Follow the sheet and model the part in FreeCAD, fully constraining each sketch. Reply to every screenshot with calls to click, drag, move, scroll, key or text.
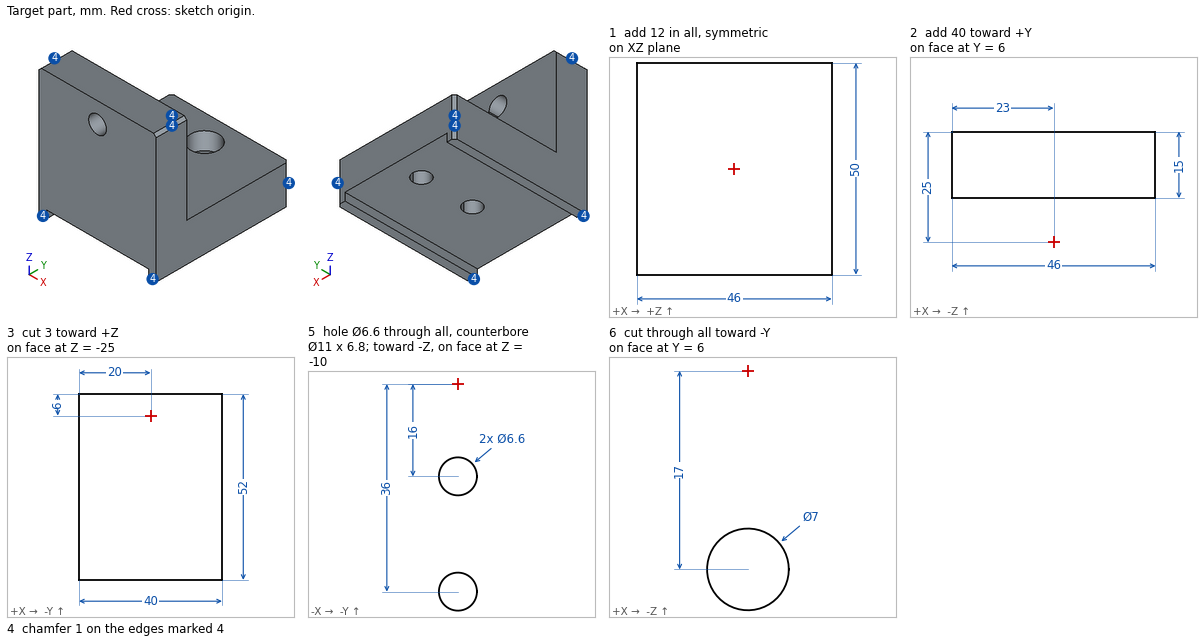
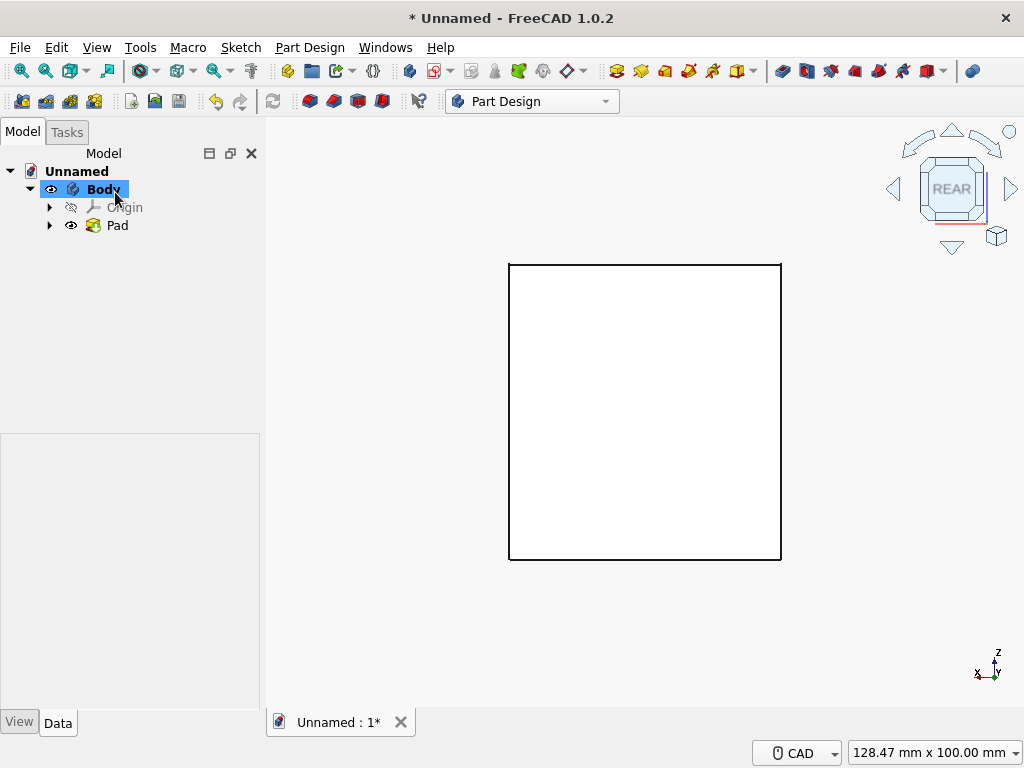
click(645, 411)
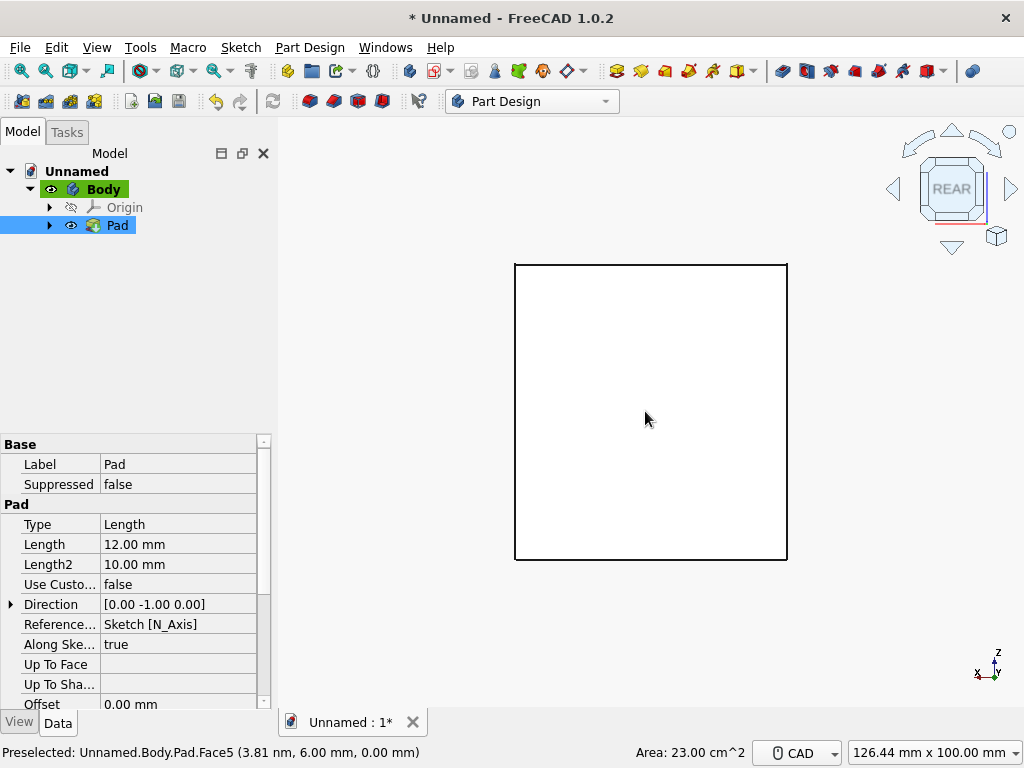
click(434, 72)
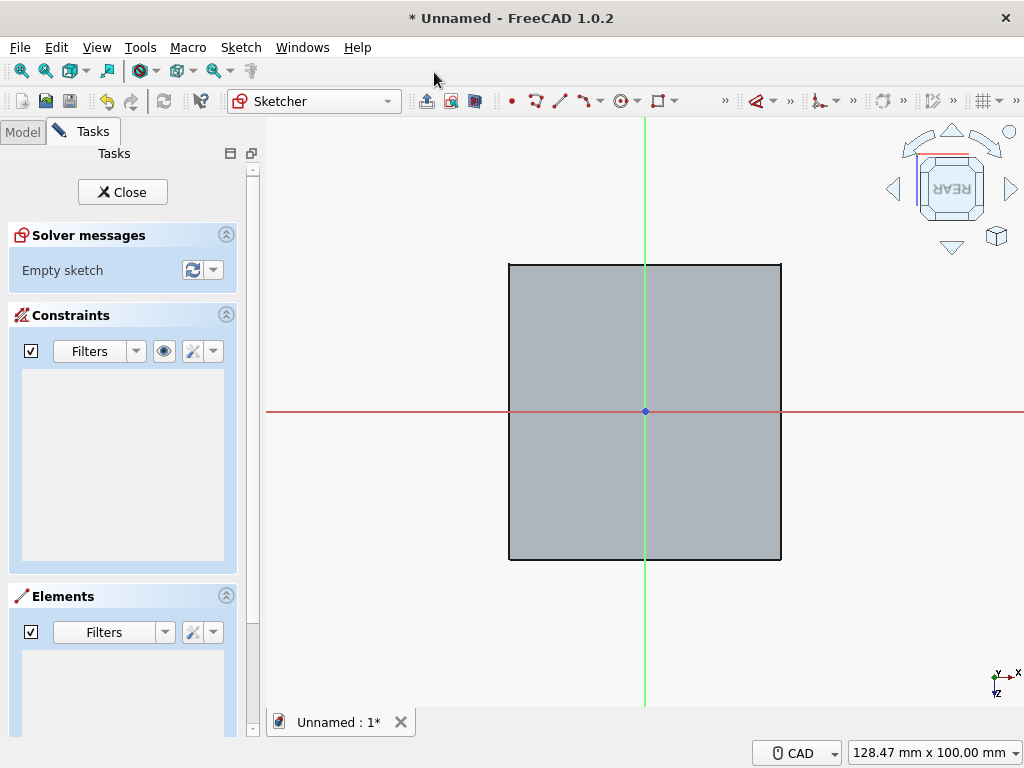
scroll(784, 188, up, 2)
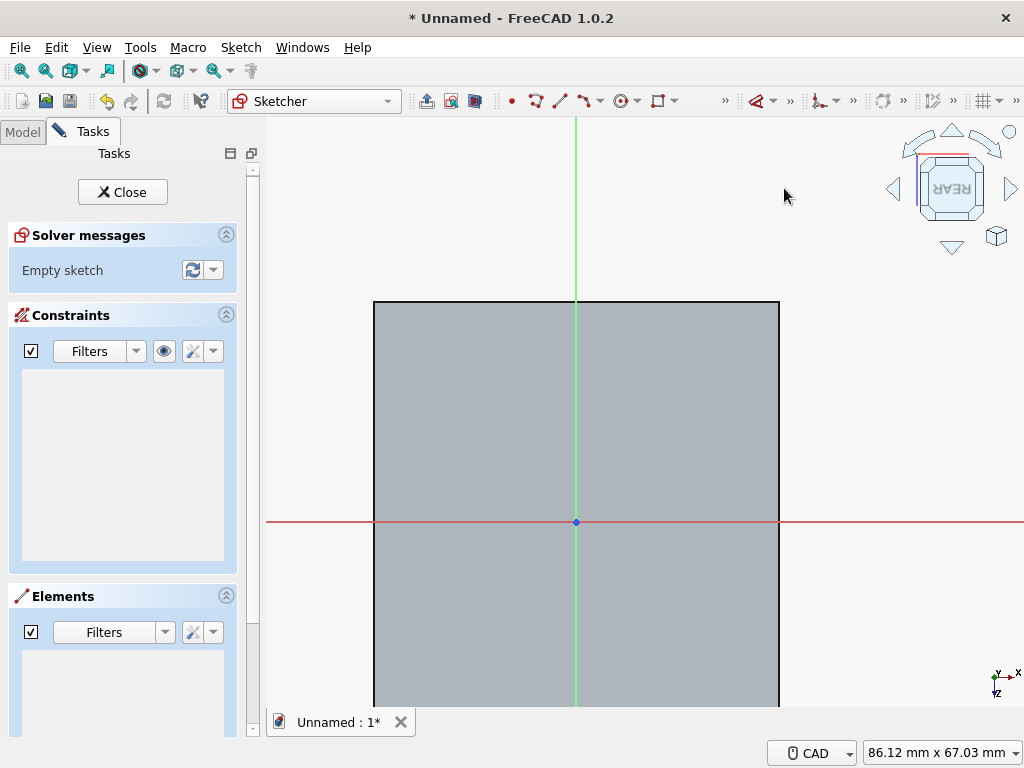
click(658, 102)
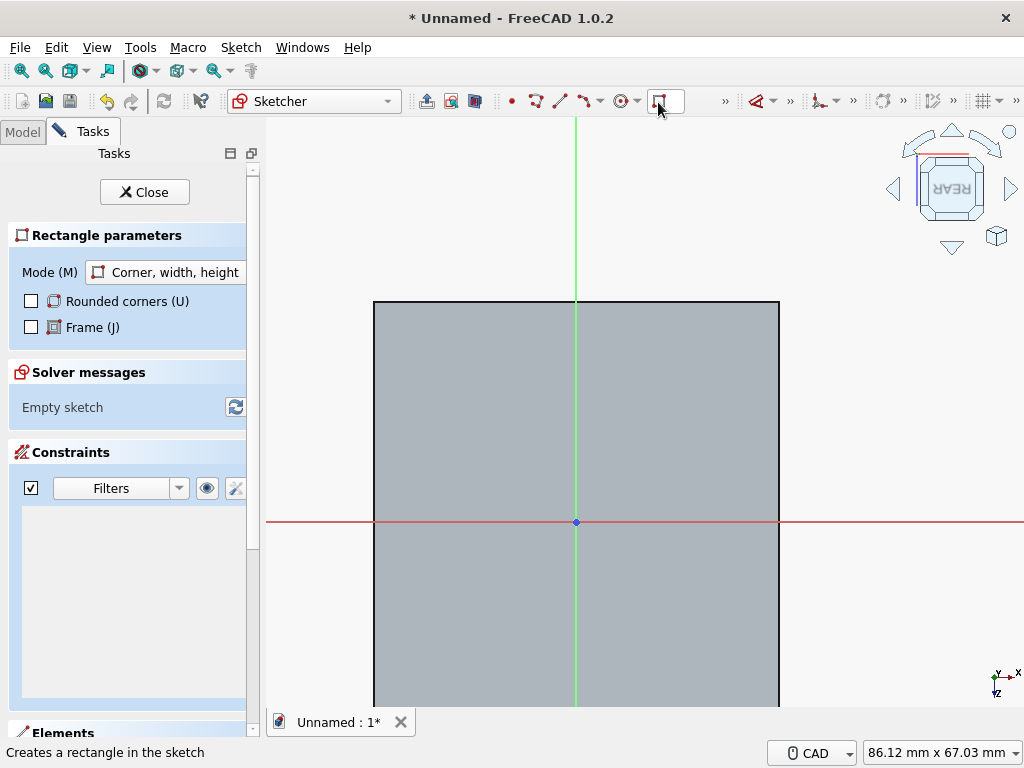
click(374, 302)
move(779, 434)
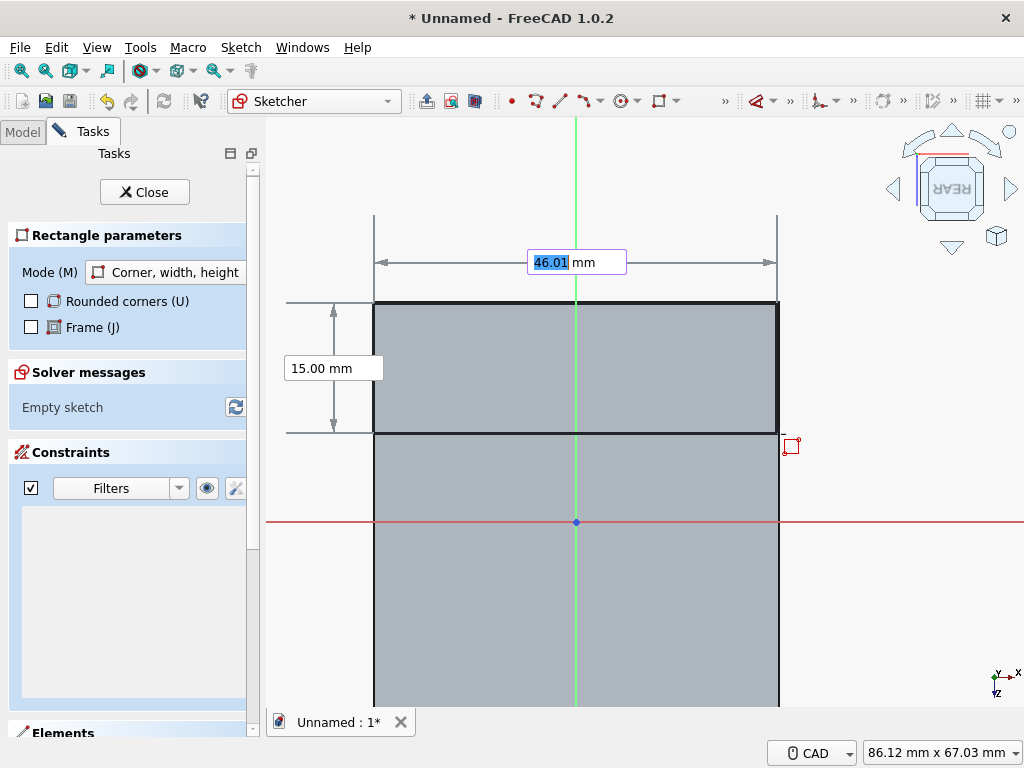
text(46)
key(Tab)
text(15)
key(Return)
key(Escape)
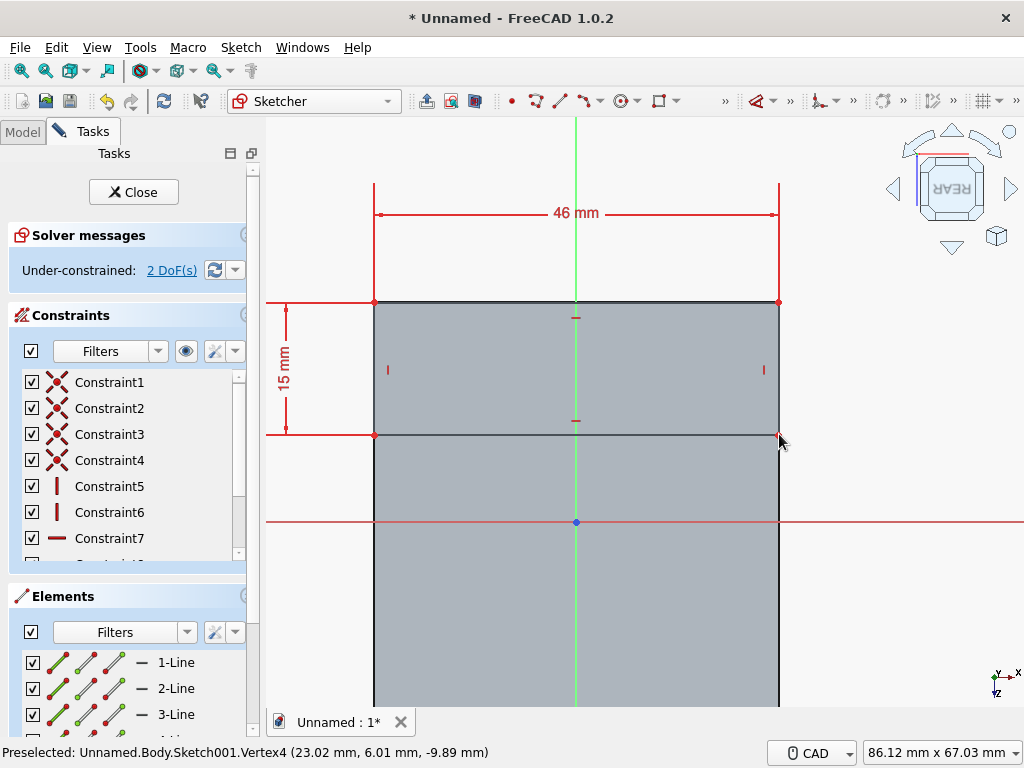
click(756, 102)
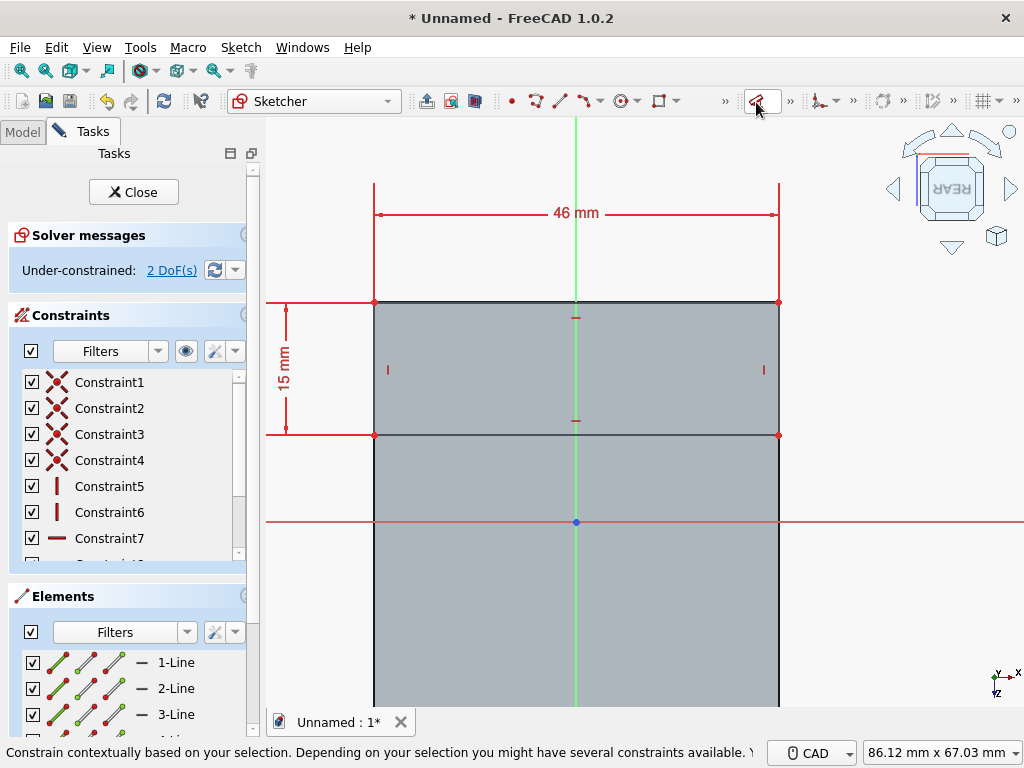
click(374, 303)
click(475, 556)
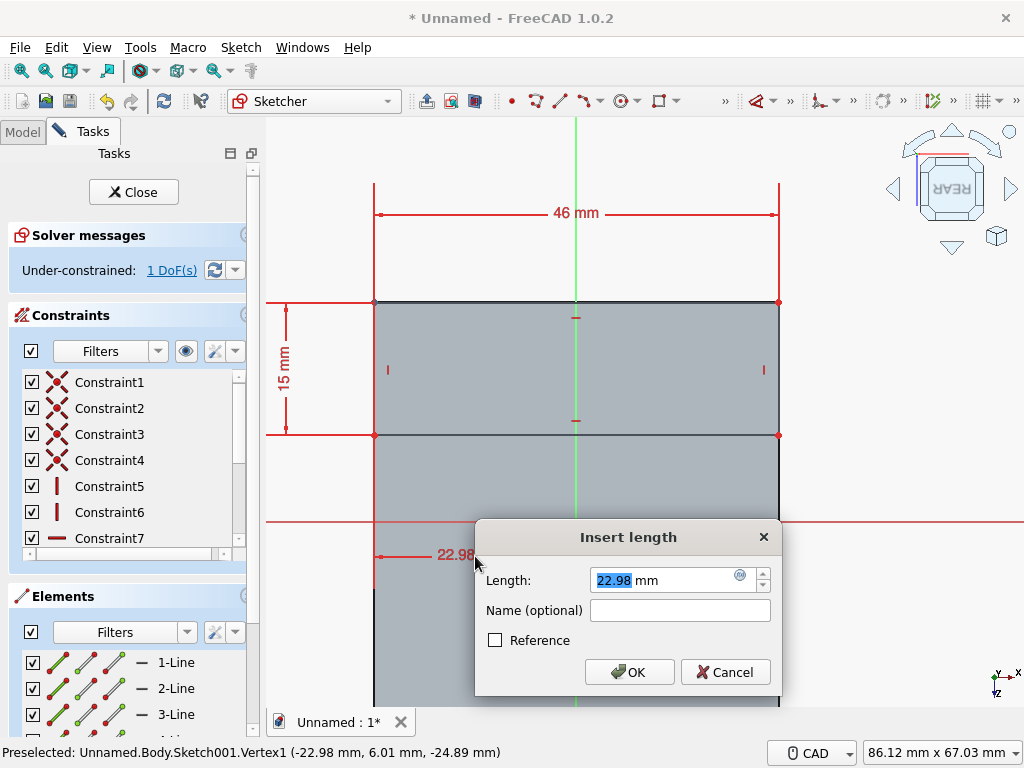
text(23)
key(Return)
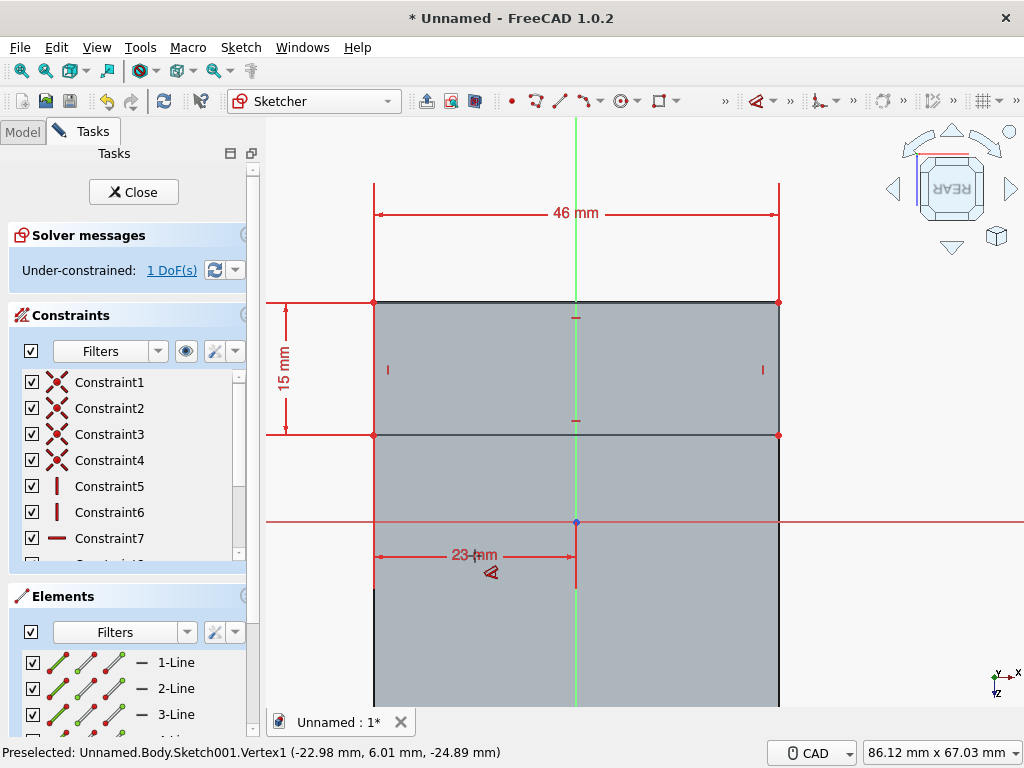
click(374, 303)
click(340, 413)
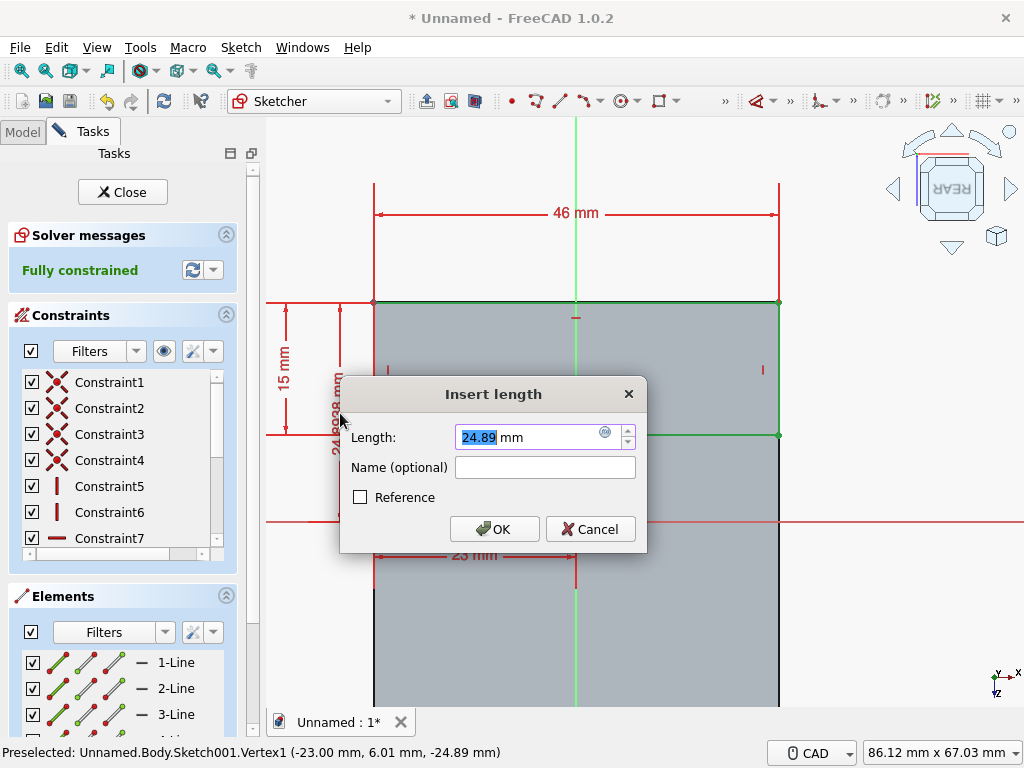
text(25)
key(Return)
key(Escape)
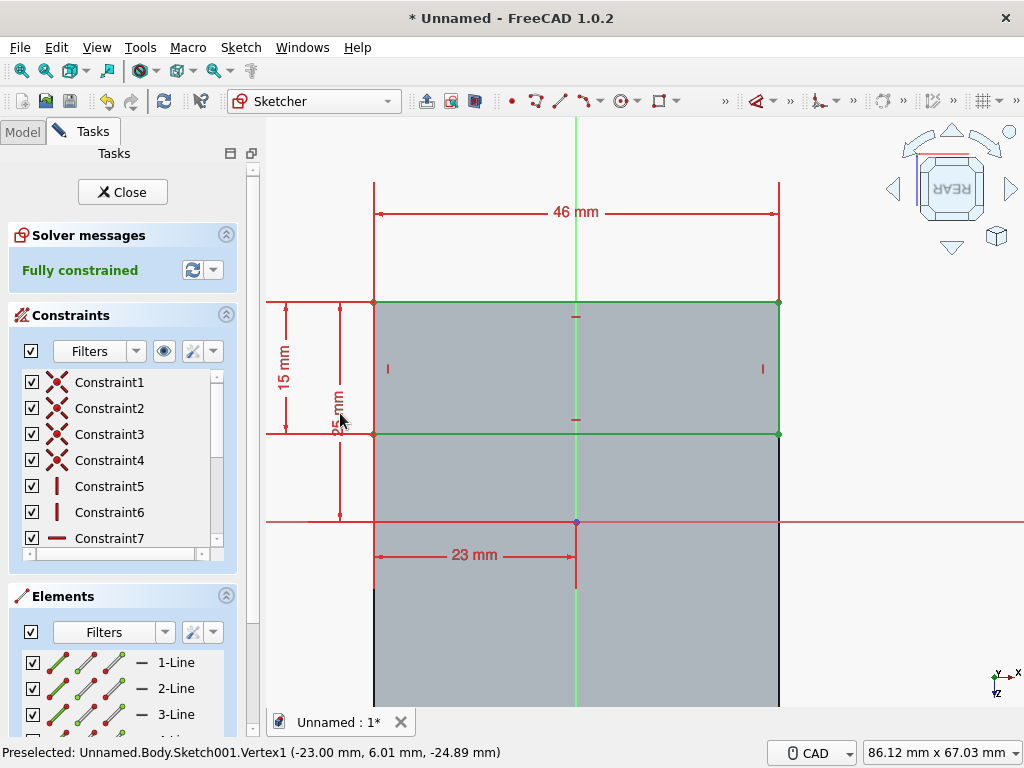
click(123, 192)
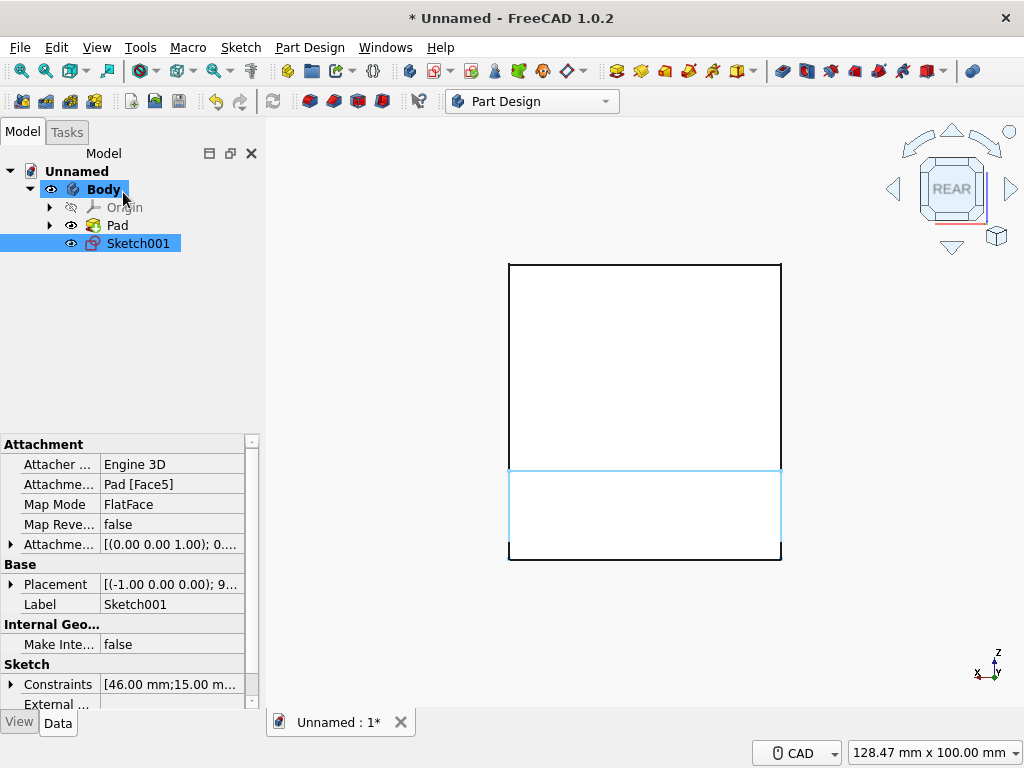
click(618, 72)